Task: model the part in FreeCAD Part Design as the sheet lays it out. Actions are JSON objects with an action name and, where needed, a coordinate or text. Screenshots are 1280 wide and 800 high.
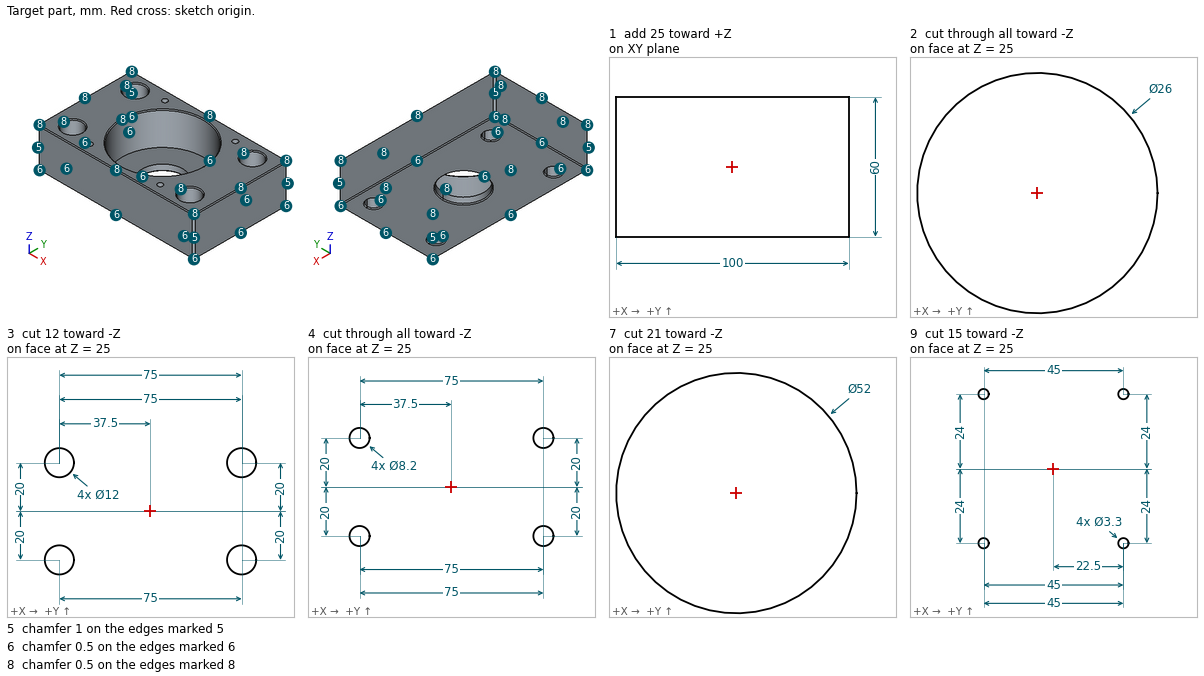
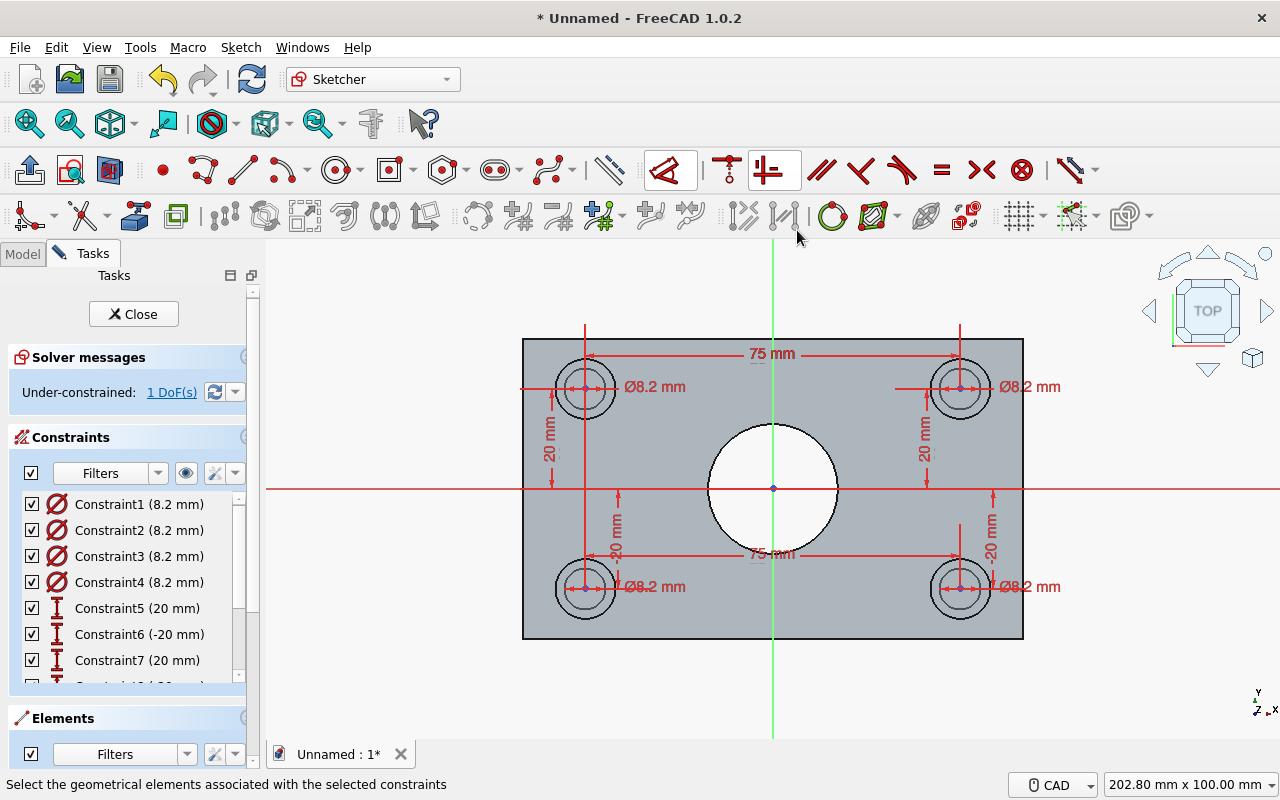
{"action": "left_click", "coordinate": [585, 389]}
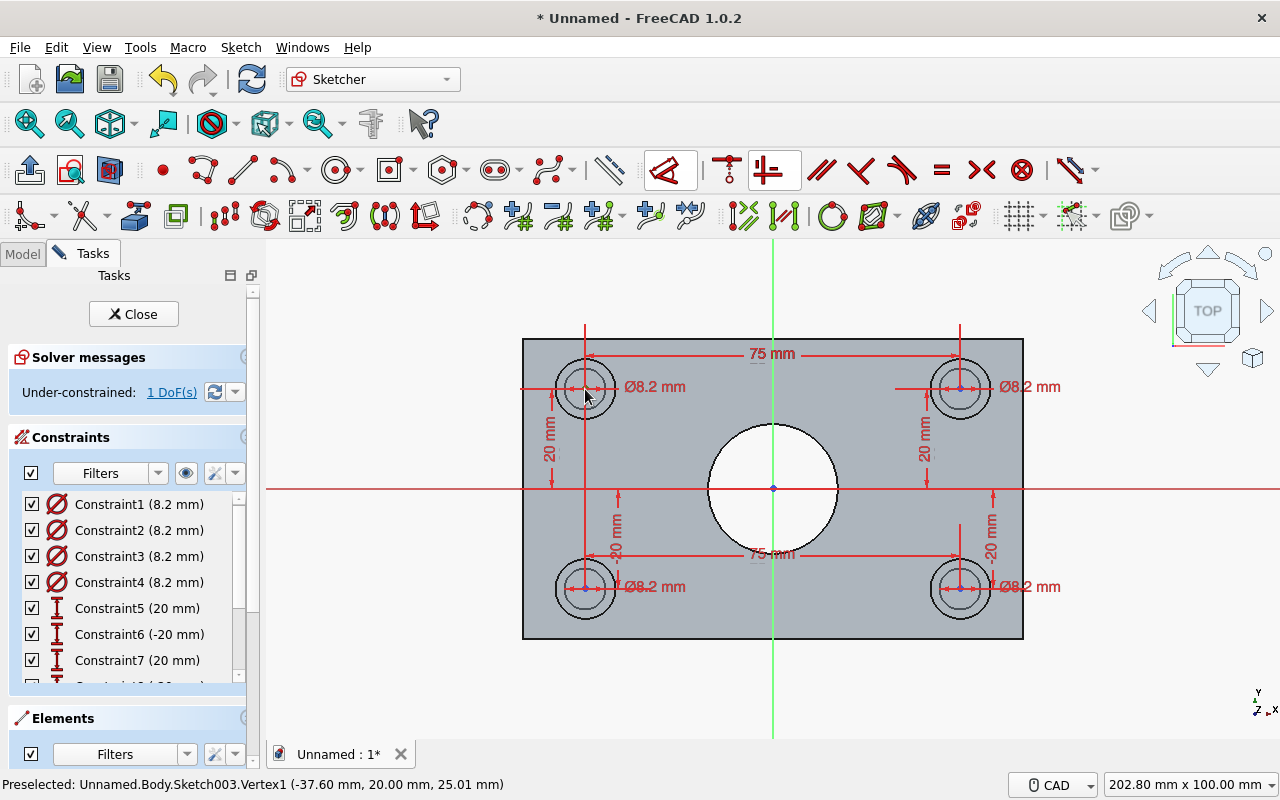
{"action": "key", "text": "l"}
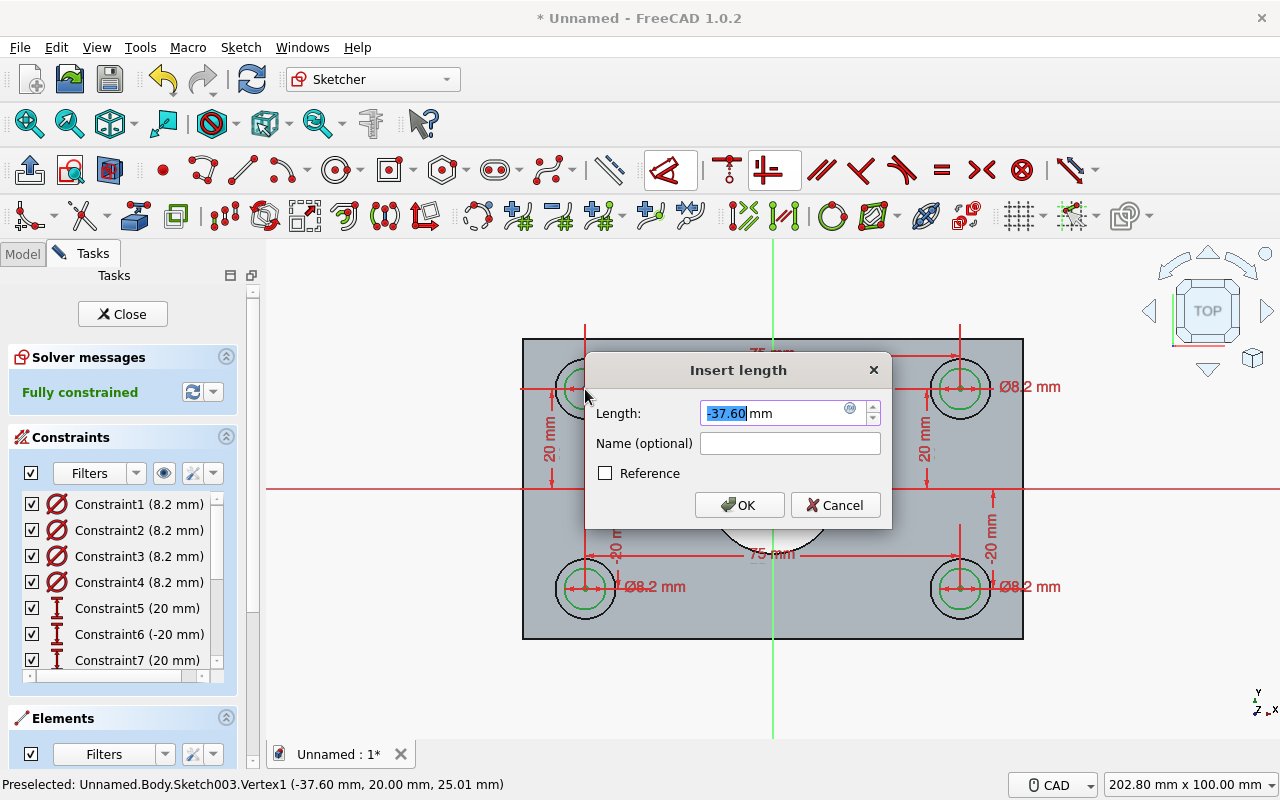
{"action": "type", "text": "-37.5"}
{"action": "key", "text": "Return"}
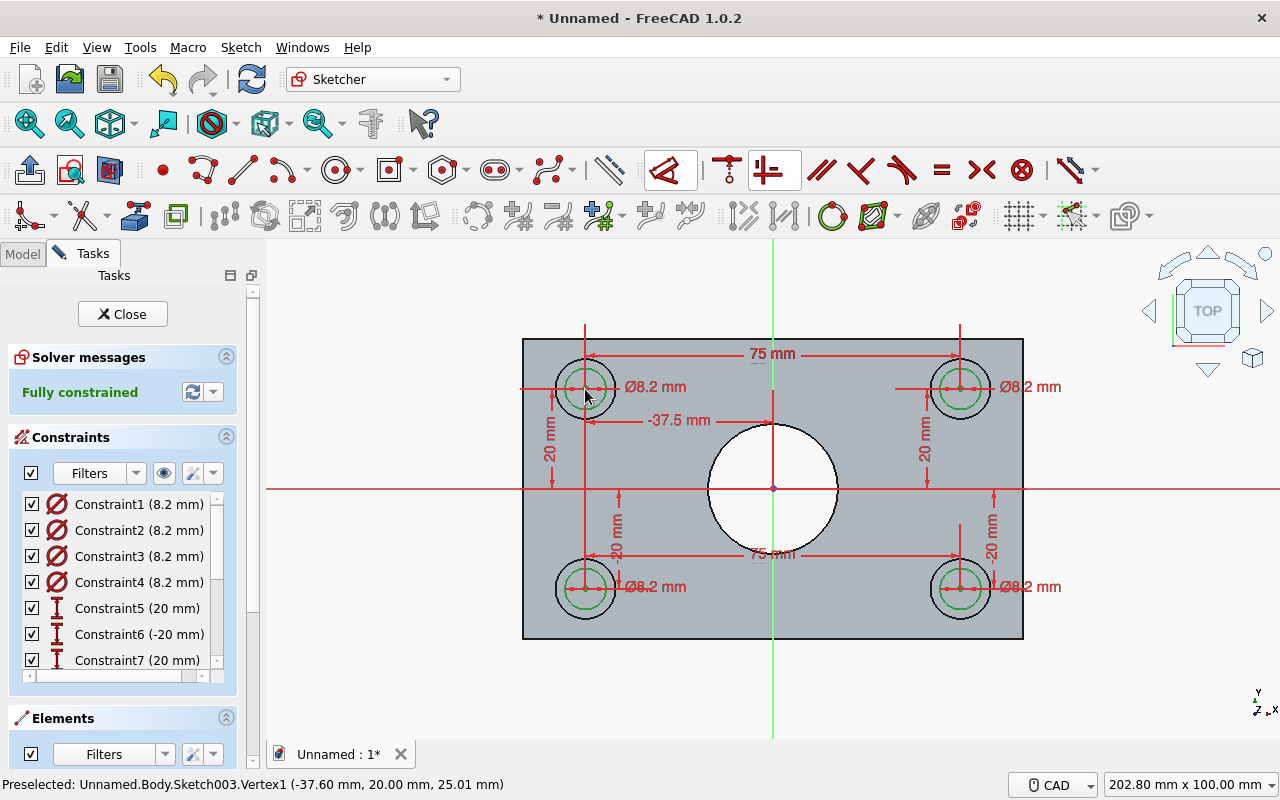
{"action": "left_click", "coordinate": [123, 314]}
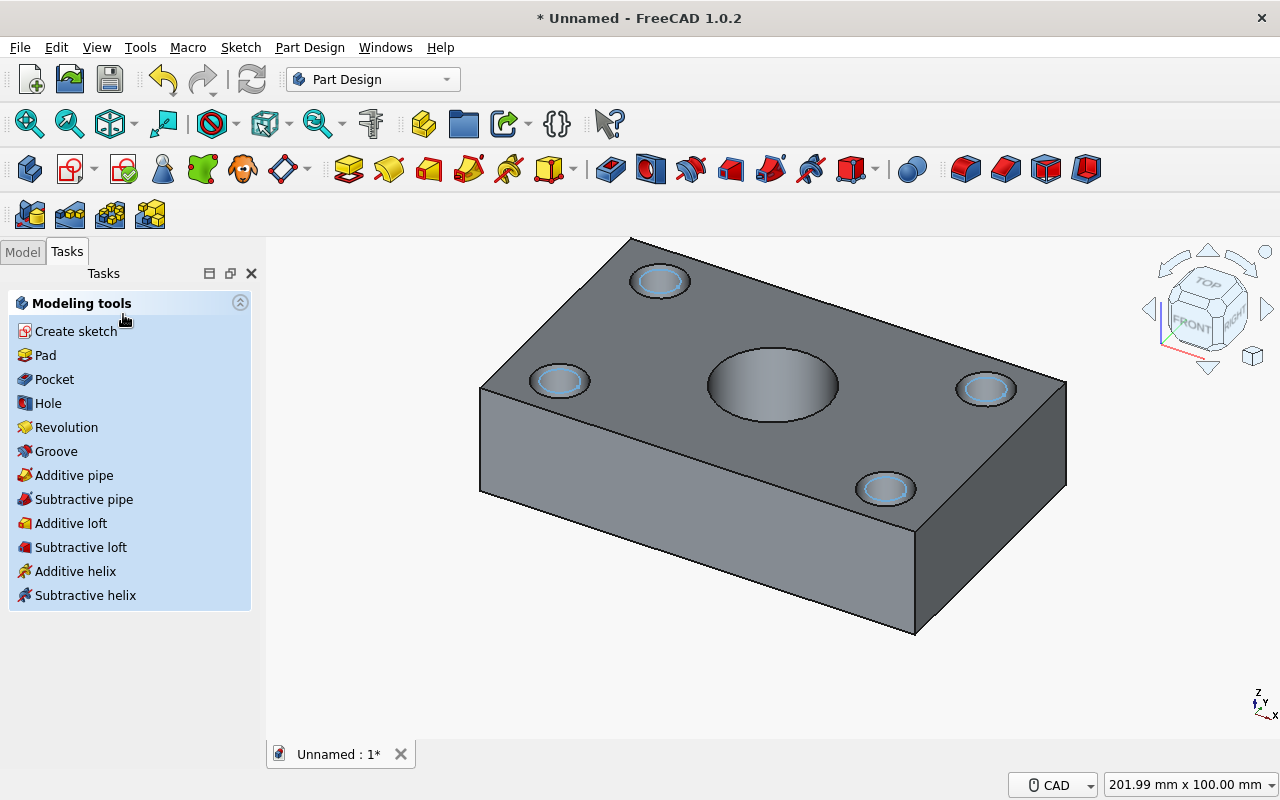
{"action": "left_click", "coordinate": [612, 170]}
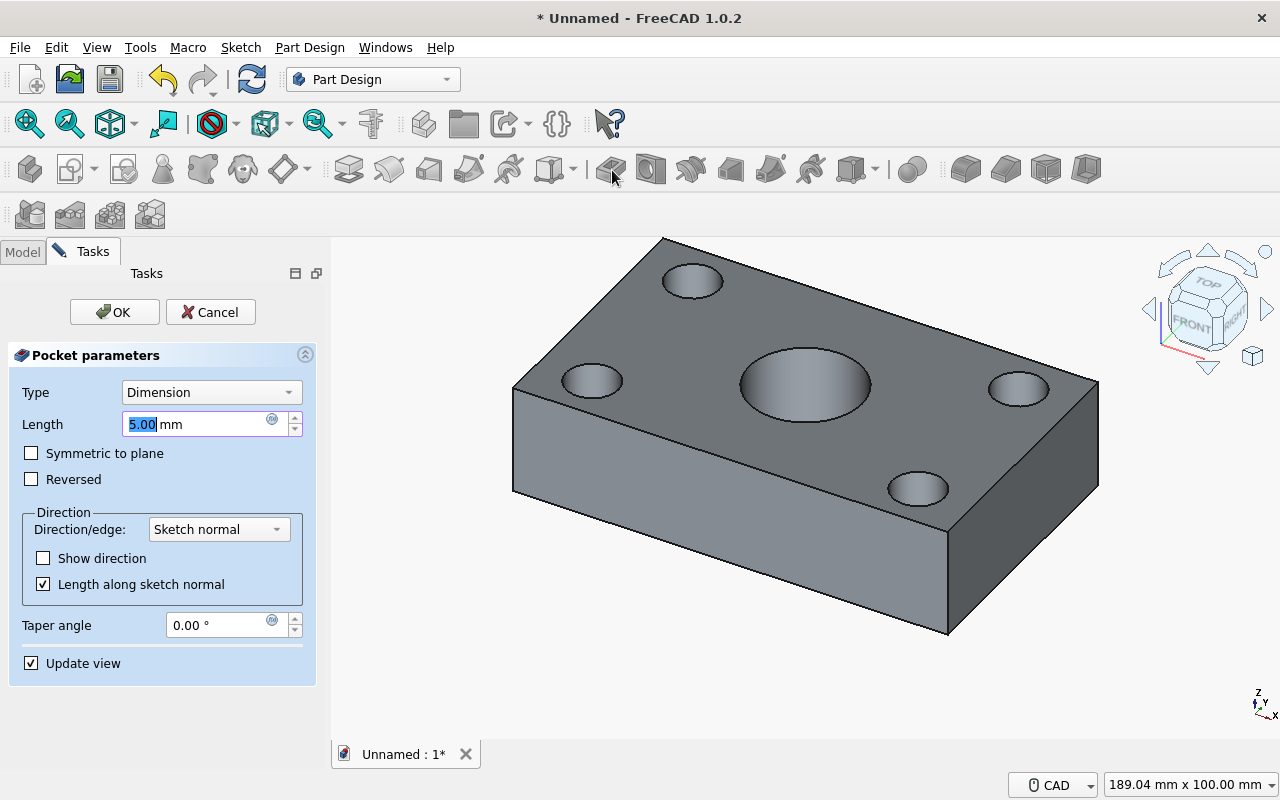
{"action": "left_click", "coordinate": [212, 392]}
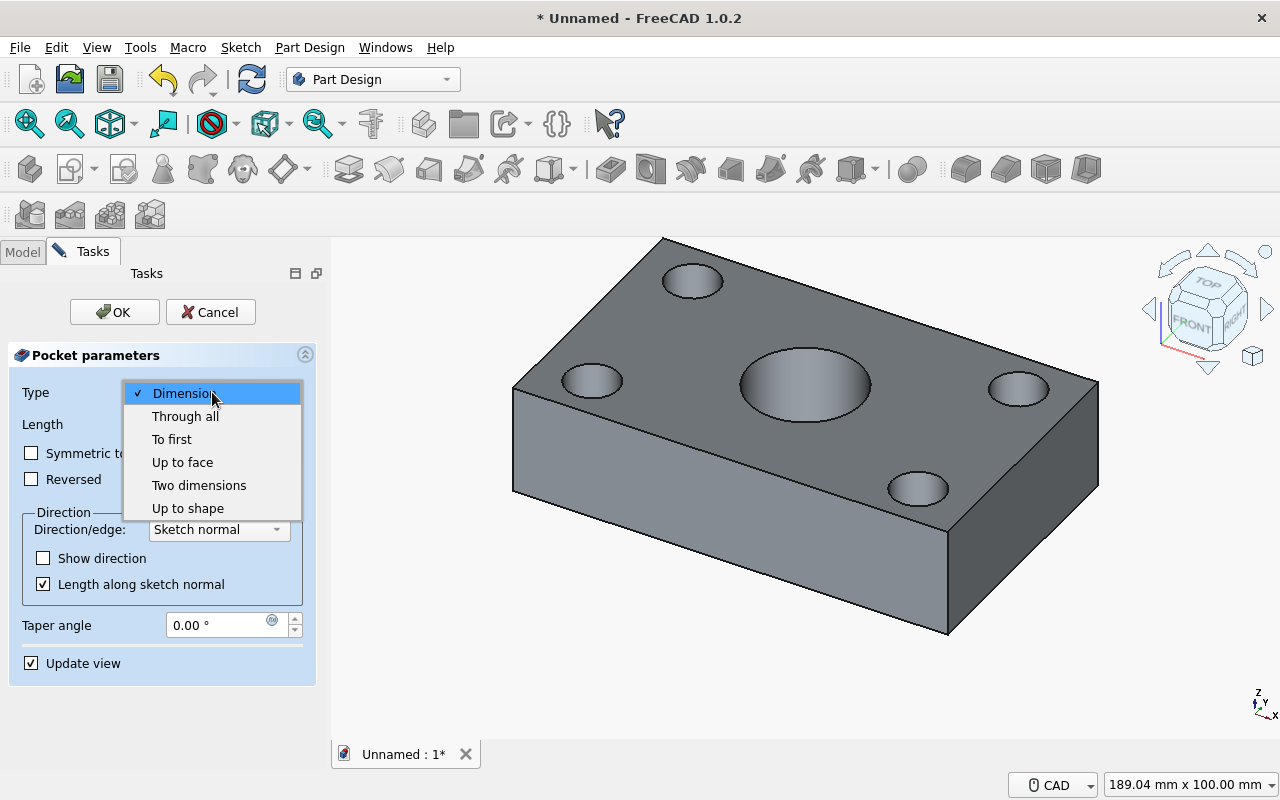
{"action": "left_click", "coordinate": [212, 416]}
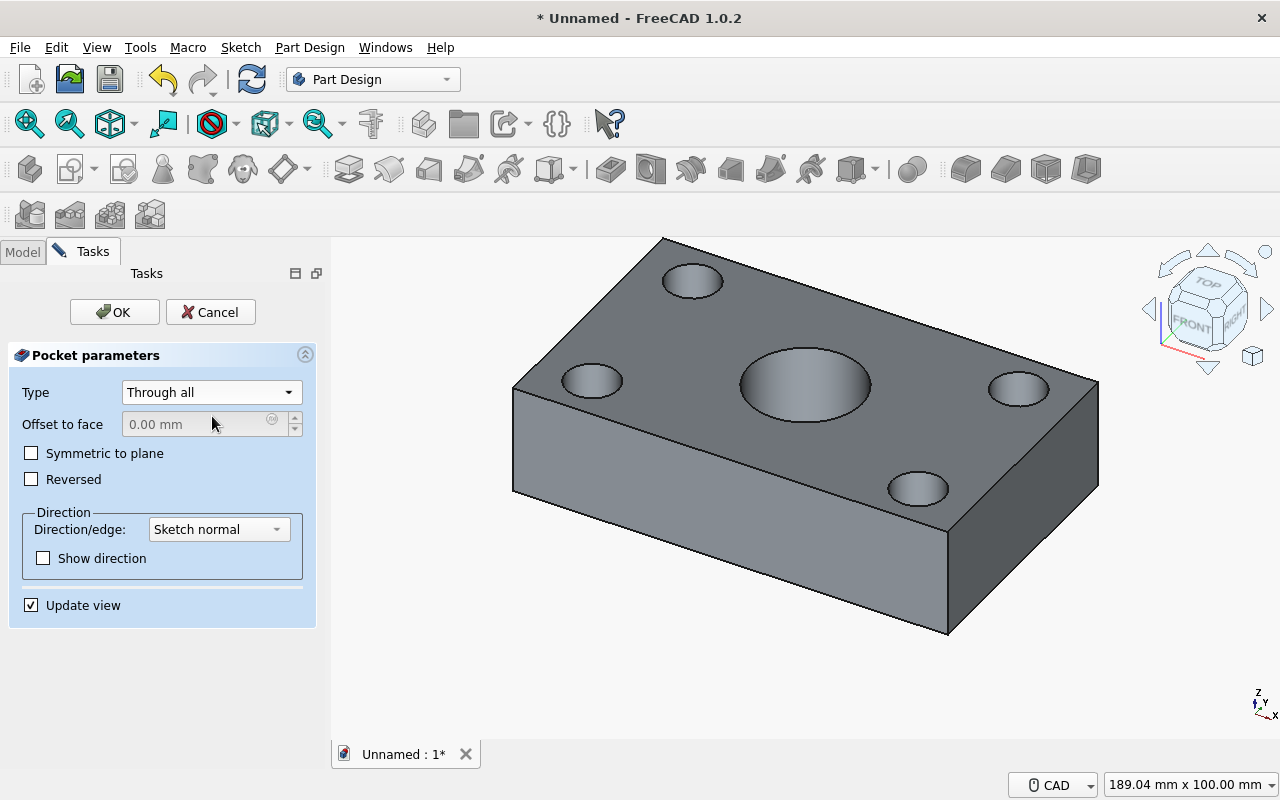
{"action": "left_click", "coordinate": [115, 312]}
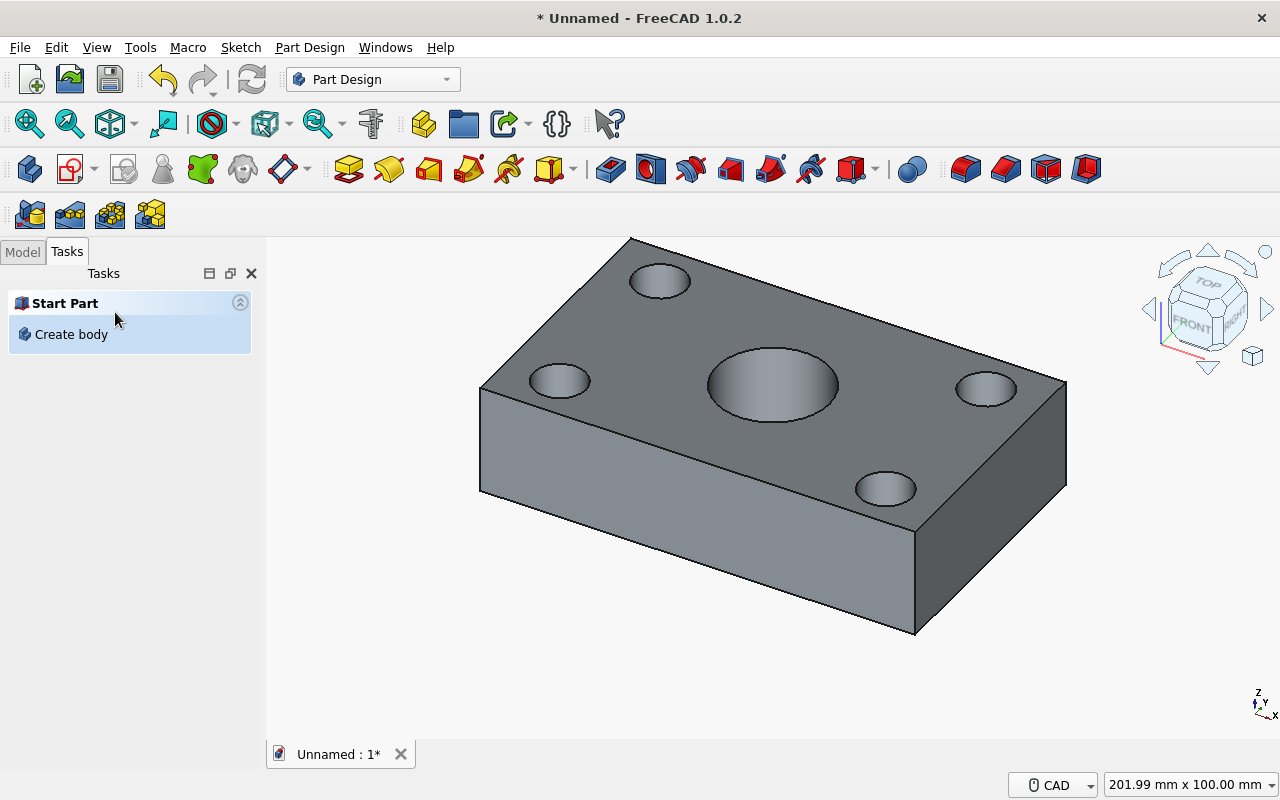
{"action": "left_click", "coordinate": [915, 582]}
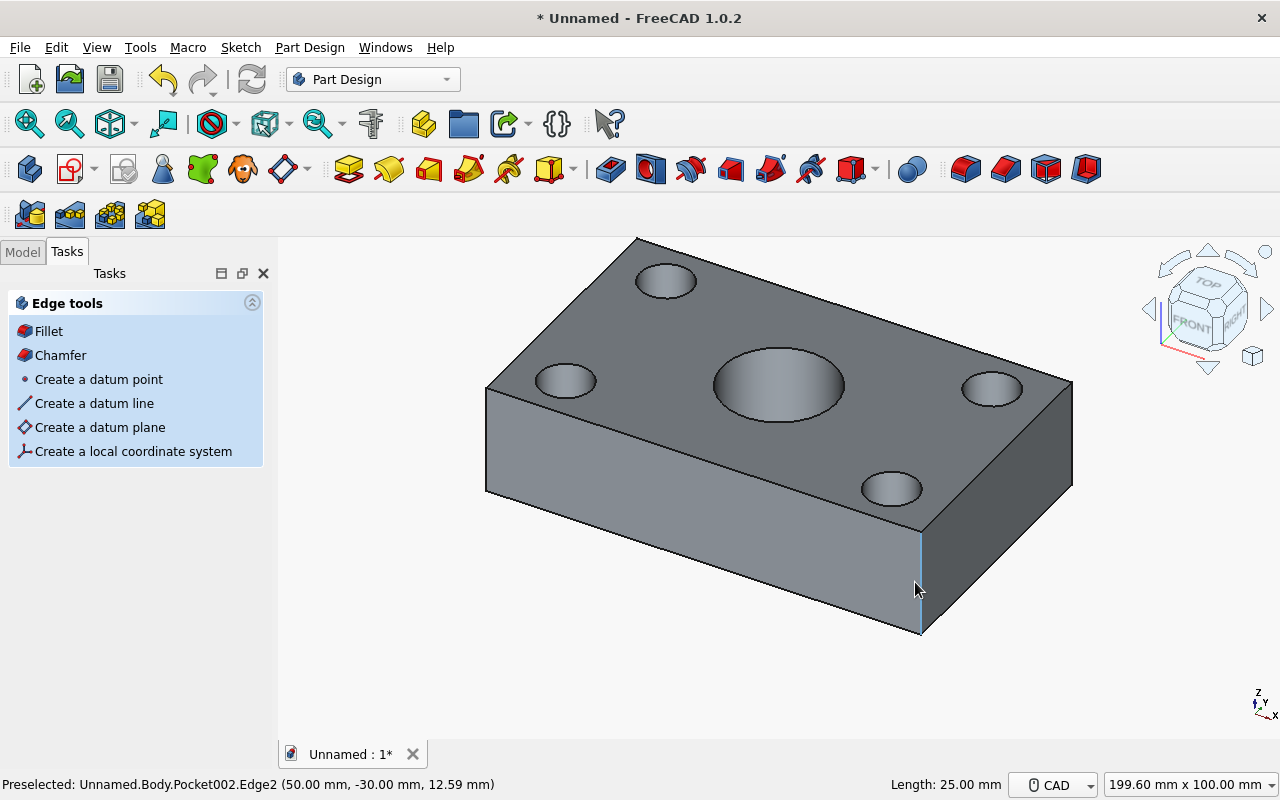
{"action": "key", "text": "0"}